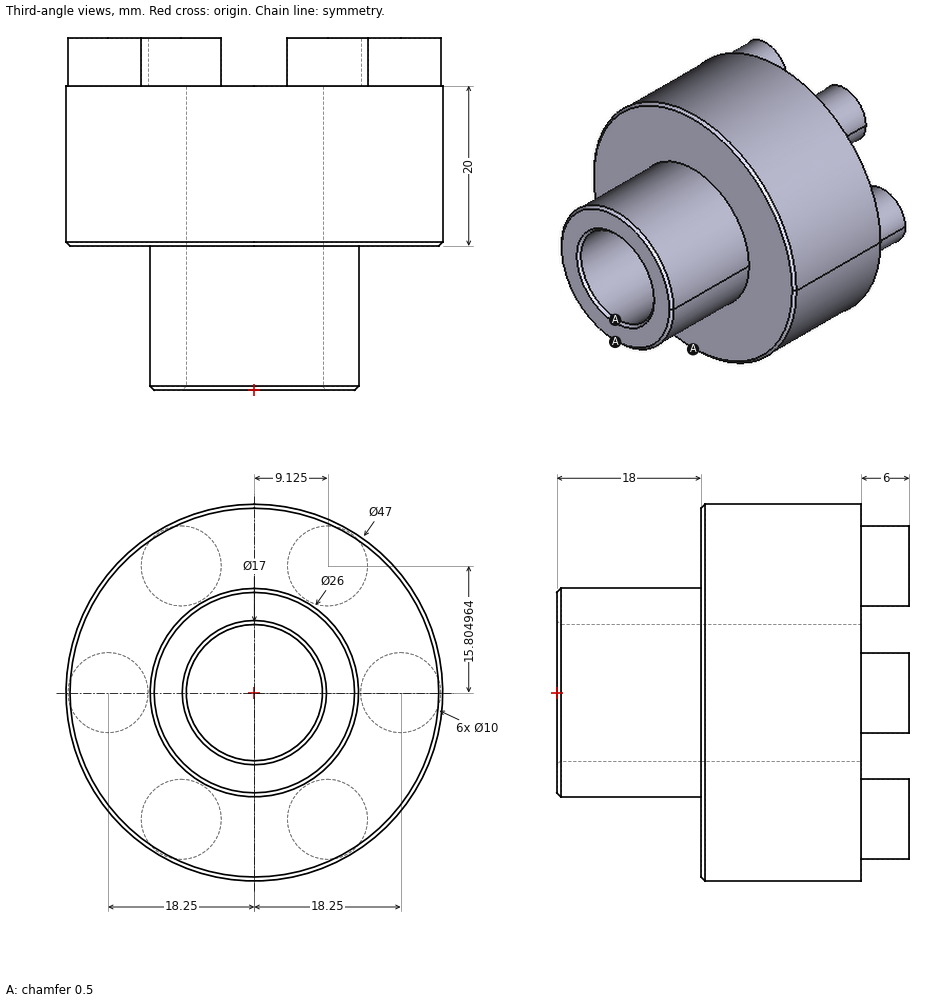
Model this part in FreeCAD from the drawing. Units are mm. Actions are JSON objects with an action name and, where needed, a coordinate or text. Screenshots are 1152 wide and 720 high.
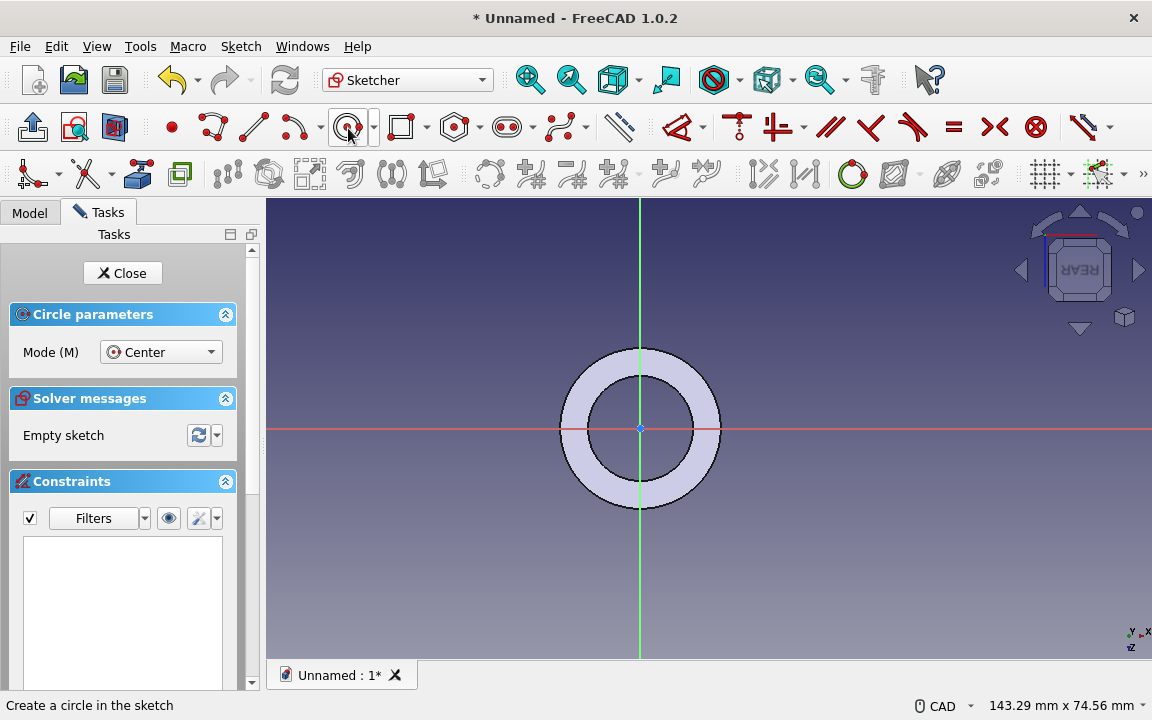
{"action": "left_click", "coordinate": [640, 429]}
{"action": "left_click", "coordinate": [743, 326]}
{"action": "key", "text": "Escape"}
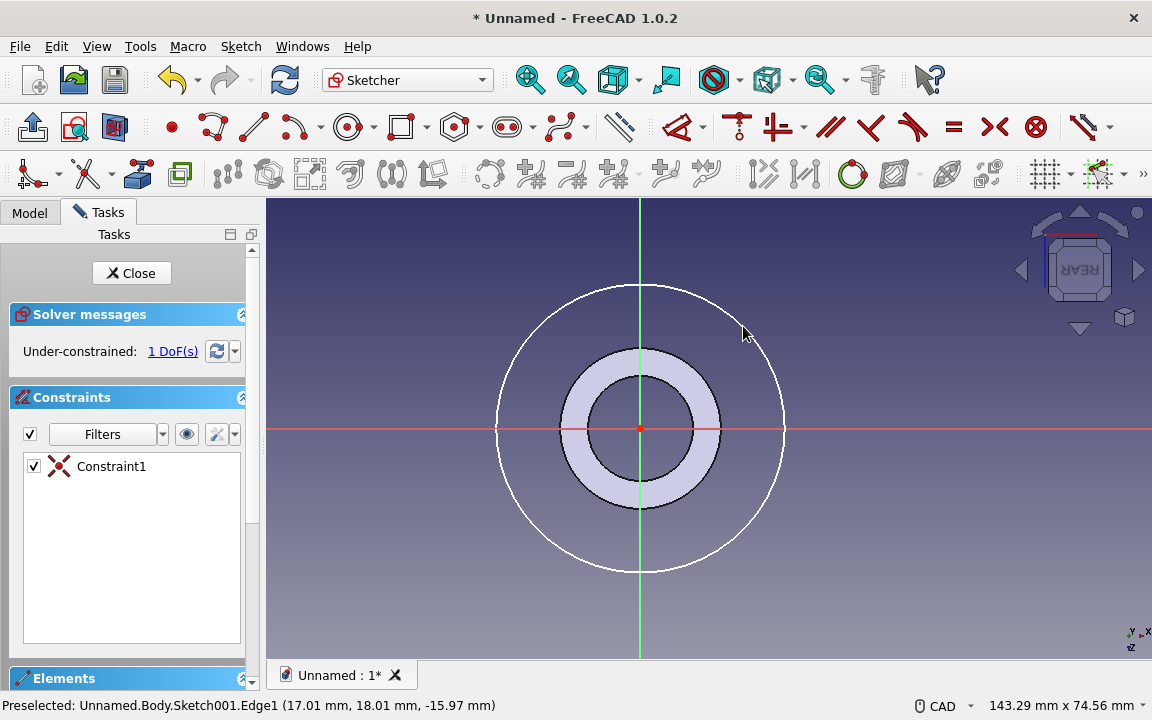
{"action": "left_click", "coordinate": [676, 128]}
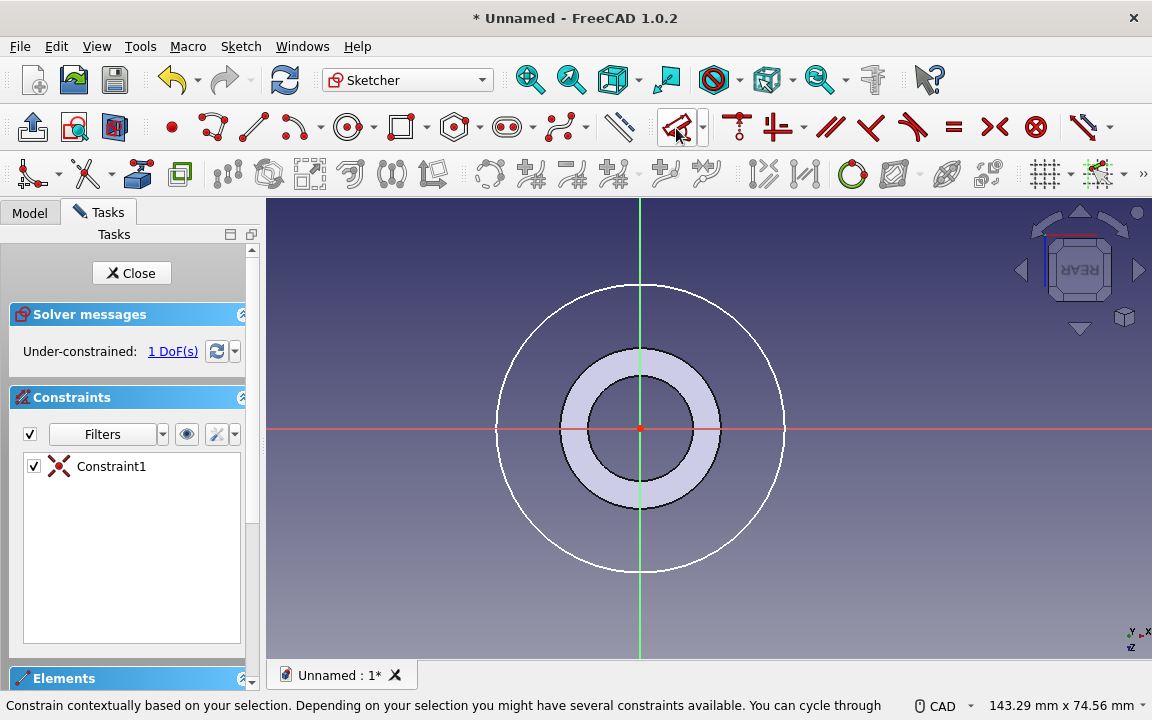
{"action": "left_click", "coordinate": [742, 326]}
{"action": "left_click", "coordinate": [765, 303]}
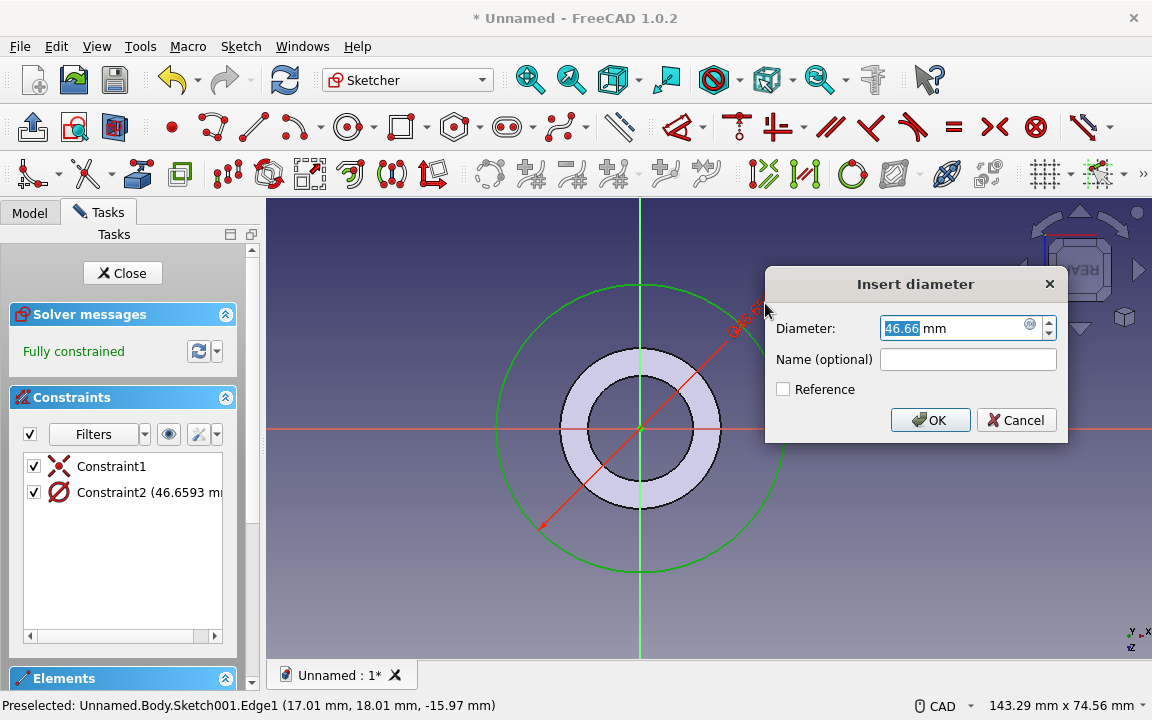
{"action": "type", "text": "47"}
{"action": "key", "text": "Return"}
{"action": "key", "text": "Escape"}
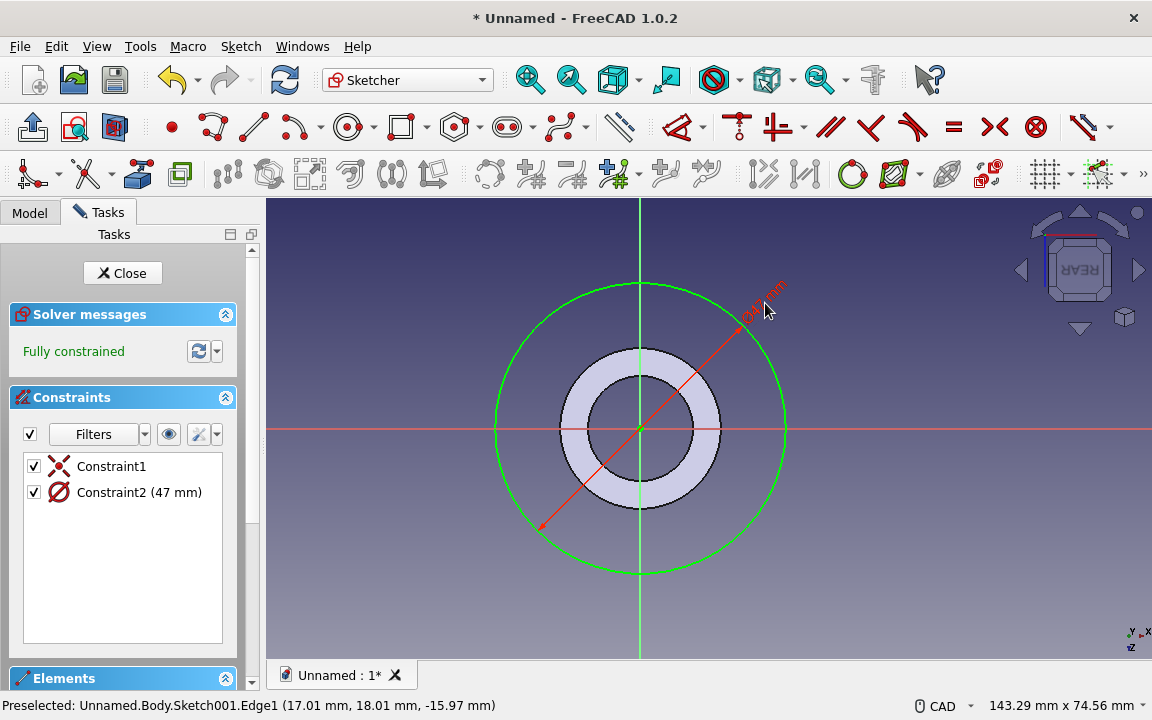
{"action": "left_click", "coordinate": [123, 273]}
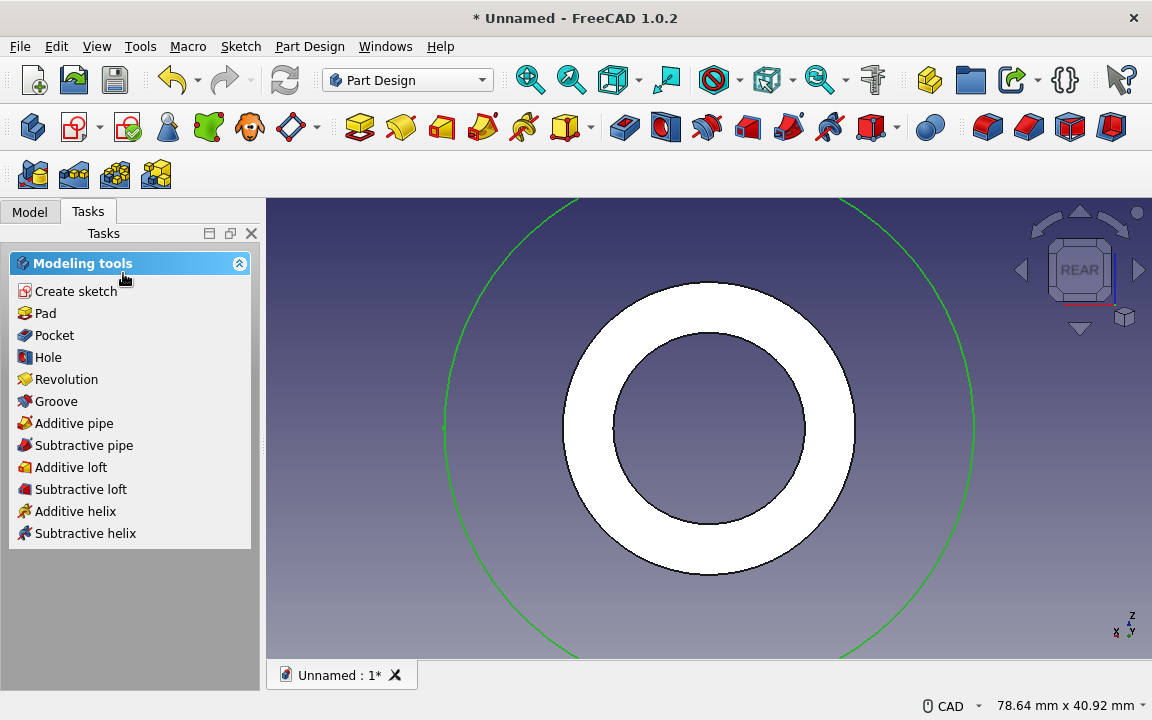
{"action": "left_click", "coordinate": [360, 128]}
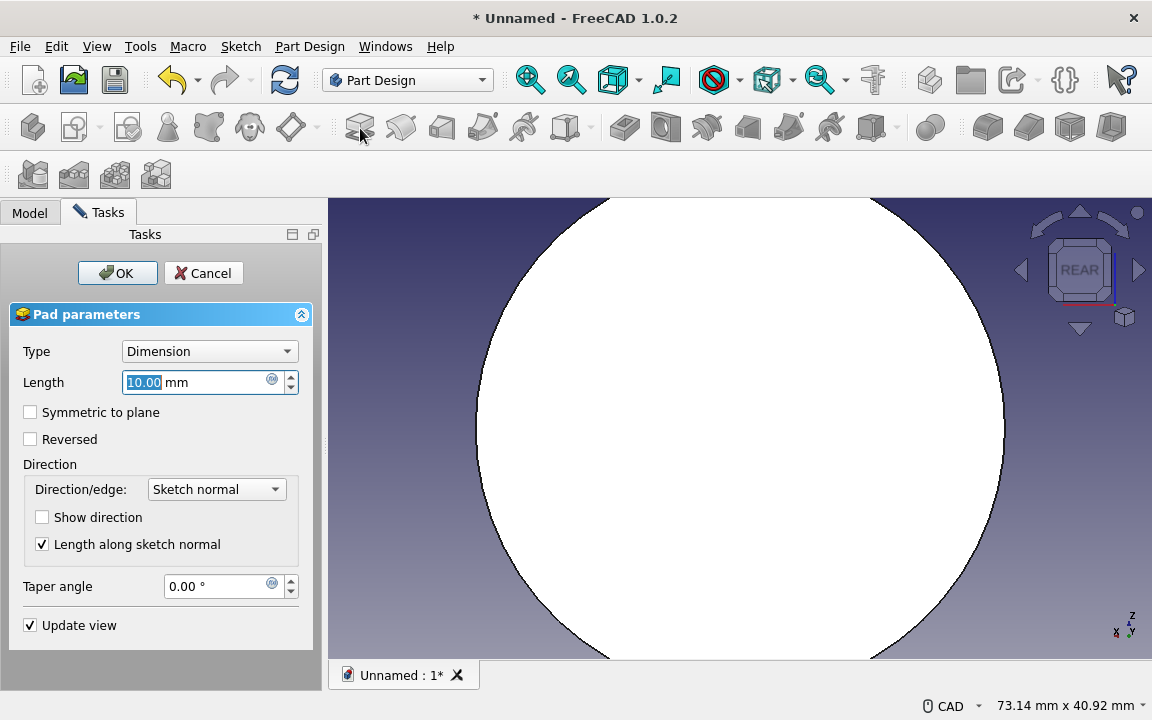
{"action": "type", "text": "20"}
{"action": "key", "text": "Tab"}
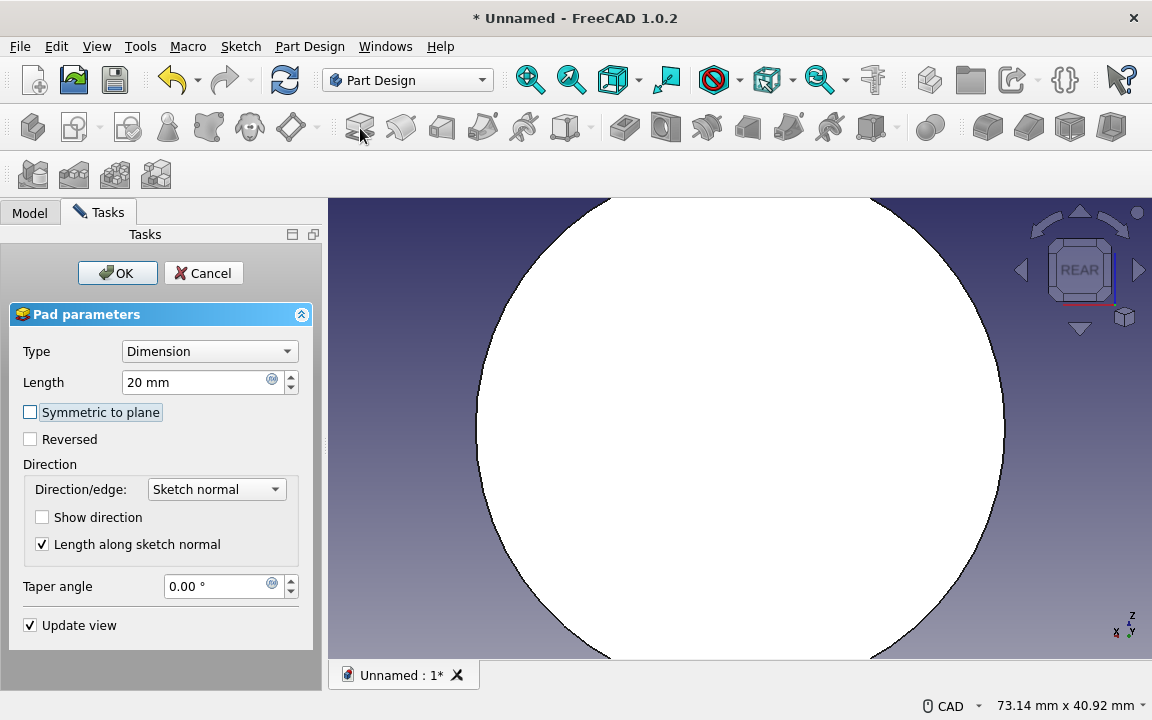
{"action": "left_click", "coordinate": [118, 273]}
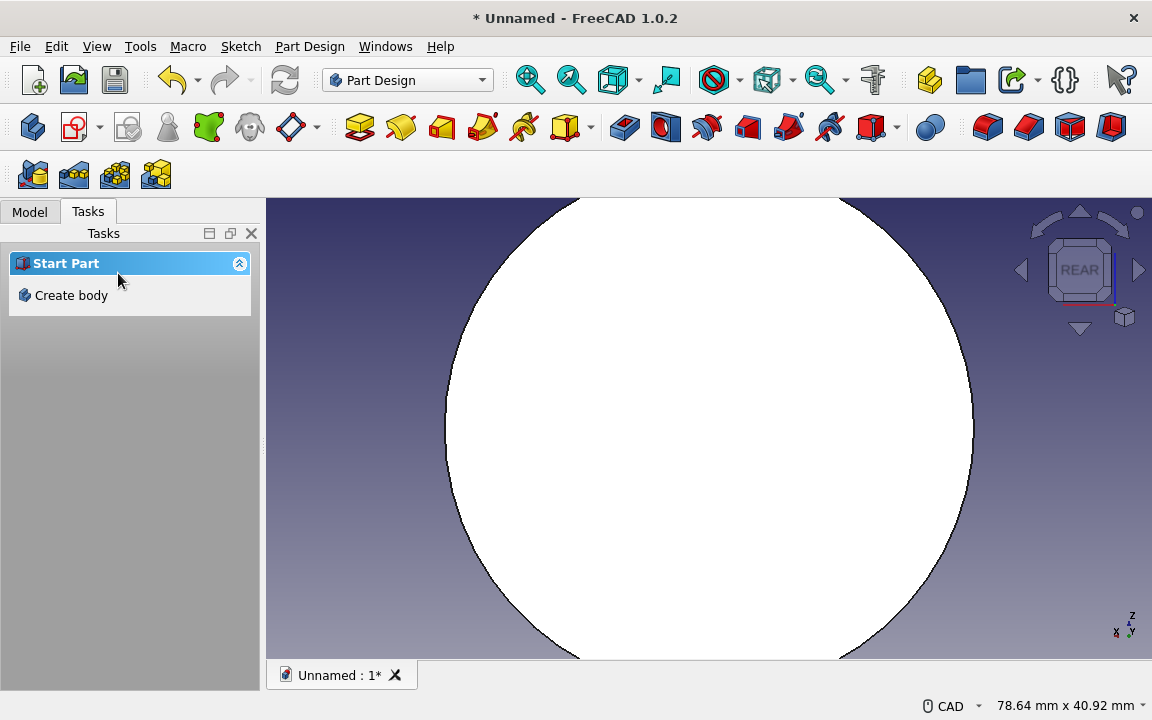
{"action": "left_click", "coordinate": [531, 80]}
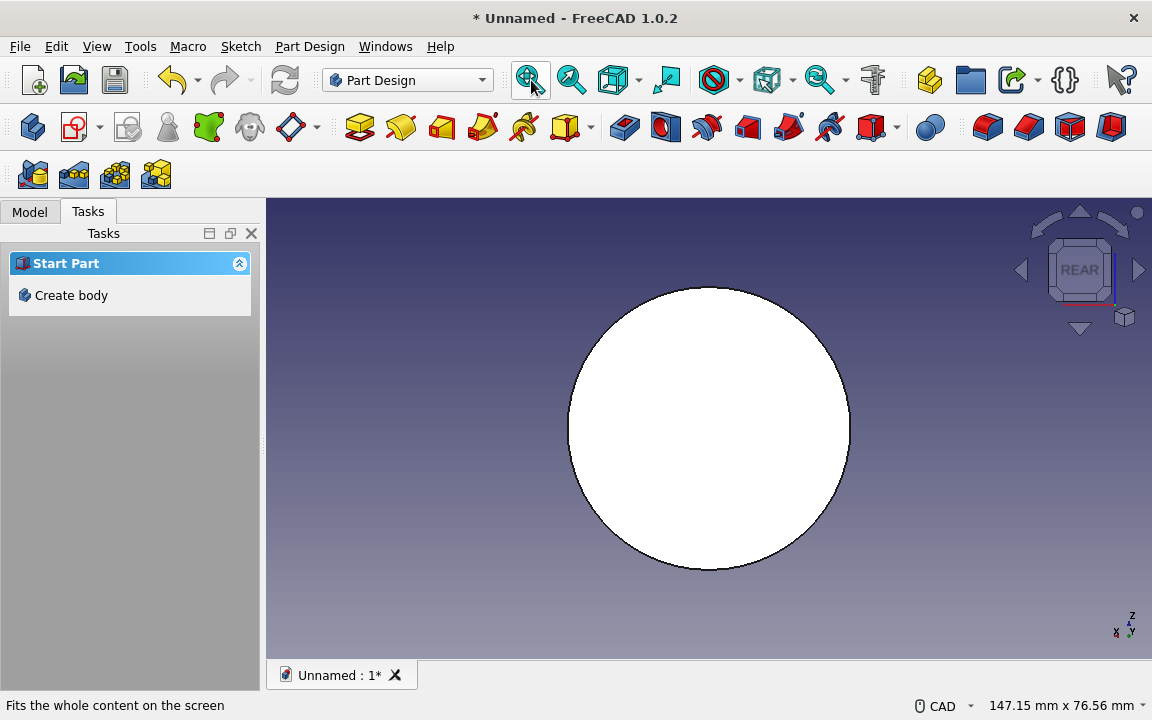
{"action": "key", "text": "0"}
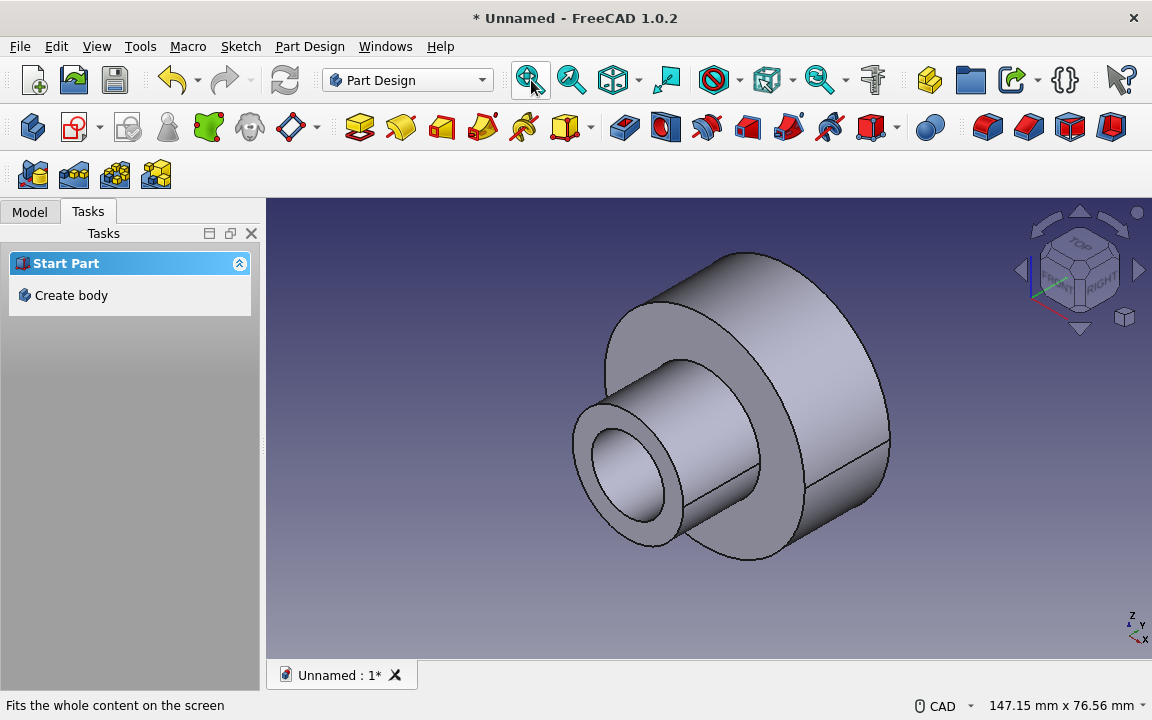
{"action": "left_click", "coordinate": [762, 529]}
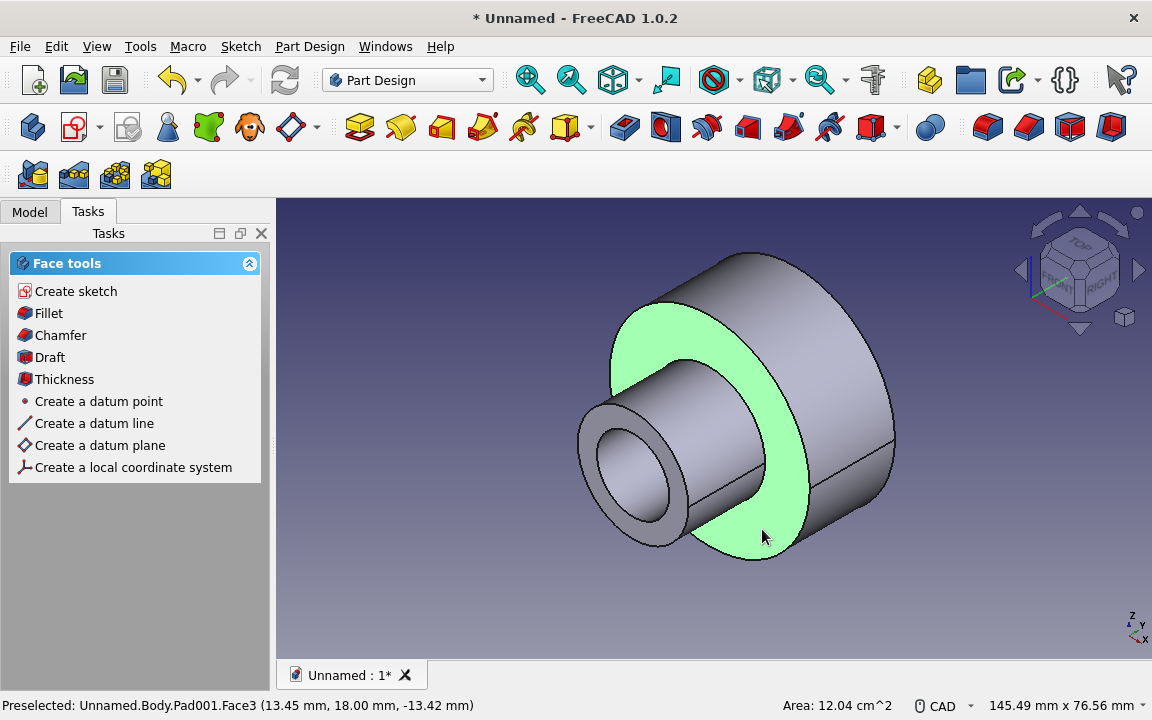
{"action": "left_click", "coordinate": [74, 128]}